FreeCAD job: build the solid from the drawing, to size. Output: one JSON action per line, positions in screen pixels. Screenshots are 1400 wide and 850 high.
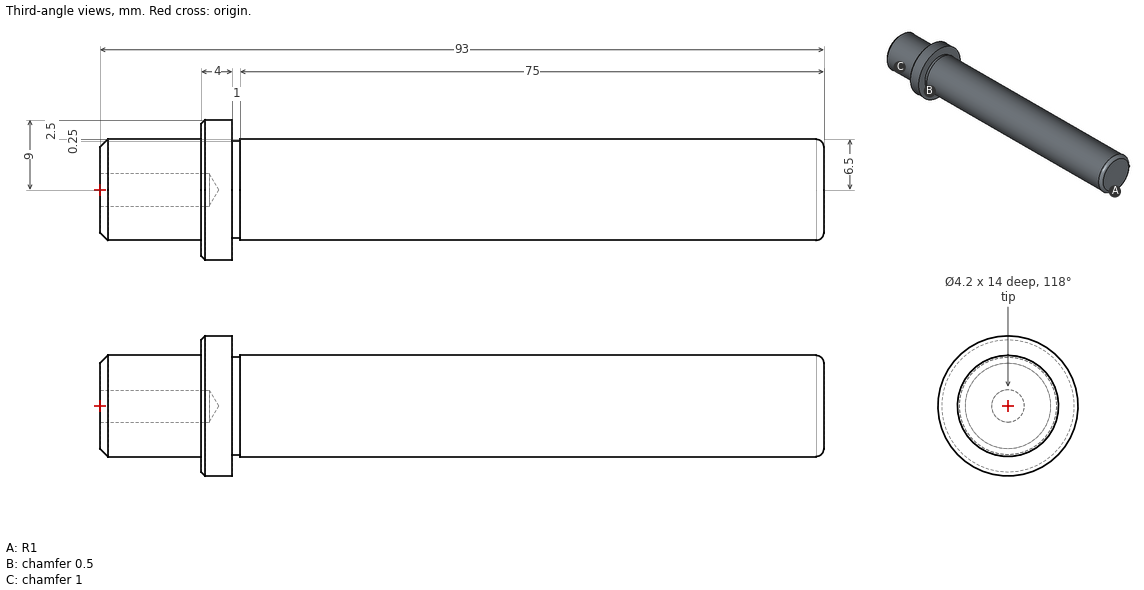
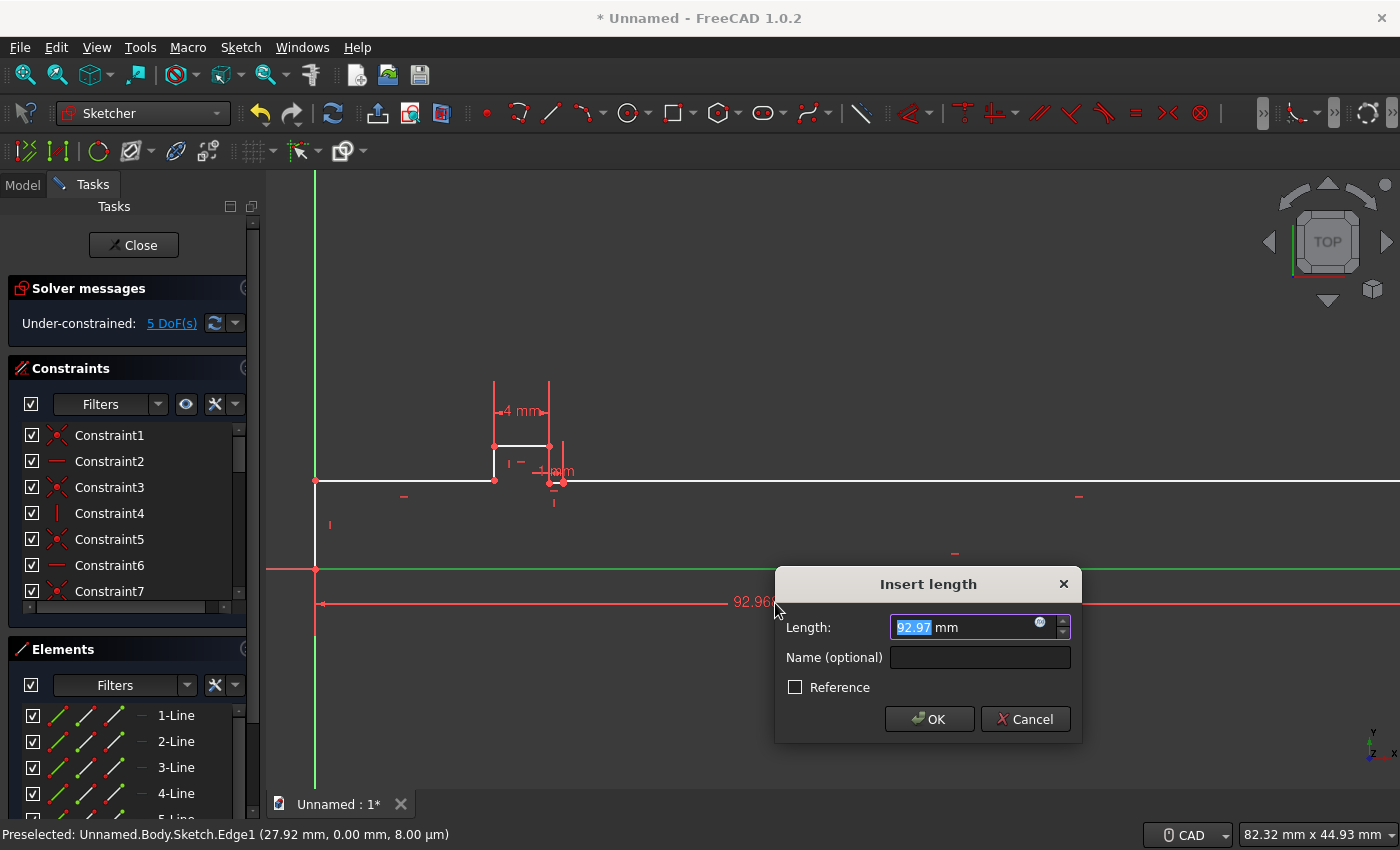
{"action": "type", "text": "93"}
{"action": "key", "text": "Return"}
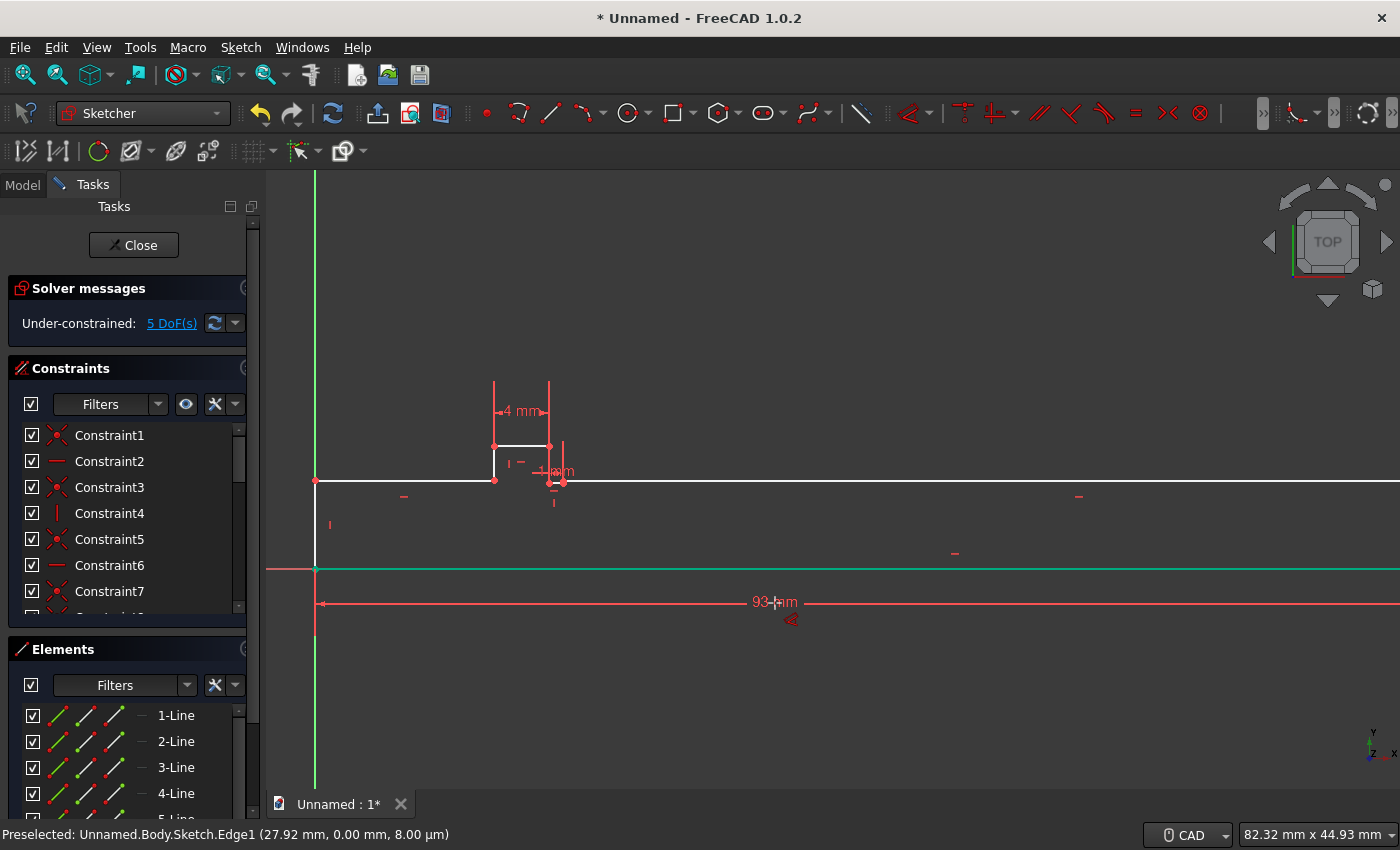
{"action": "left_click", "coordinate": [873, 481]}
{"action": "left_click", "coordinate": [899, 447]}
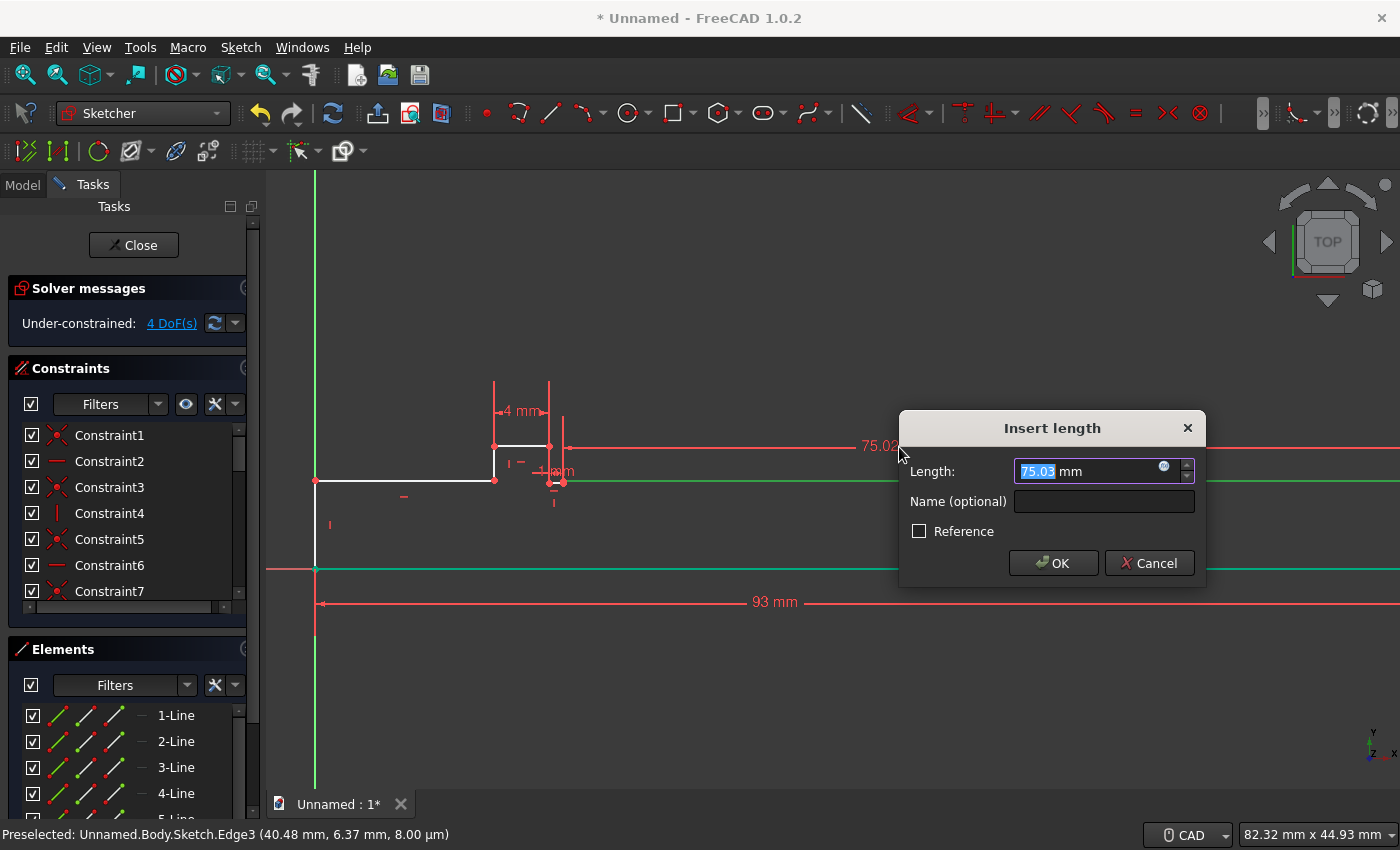
{"action": "type", "text": "75"}
{"action": "key", "text": "Return"}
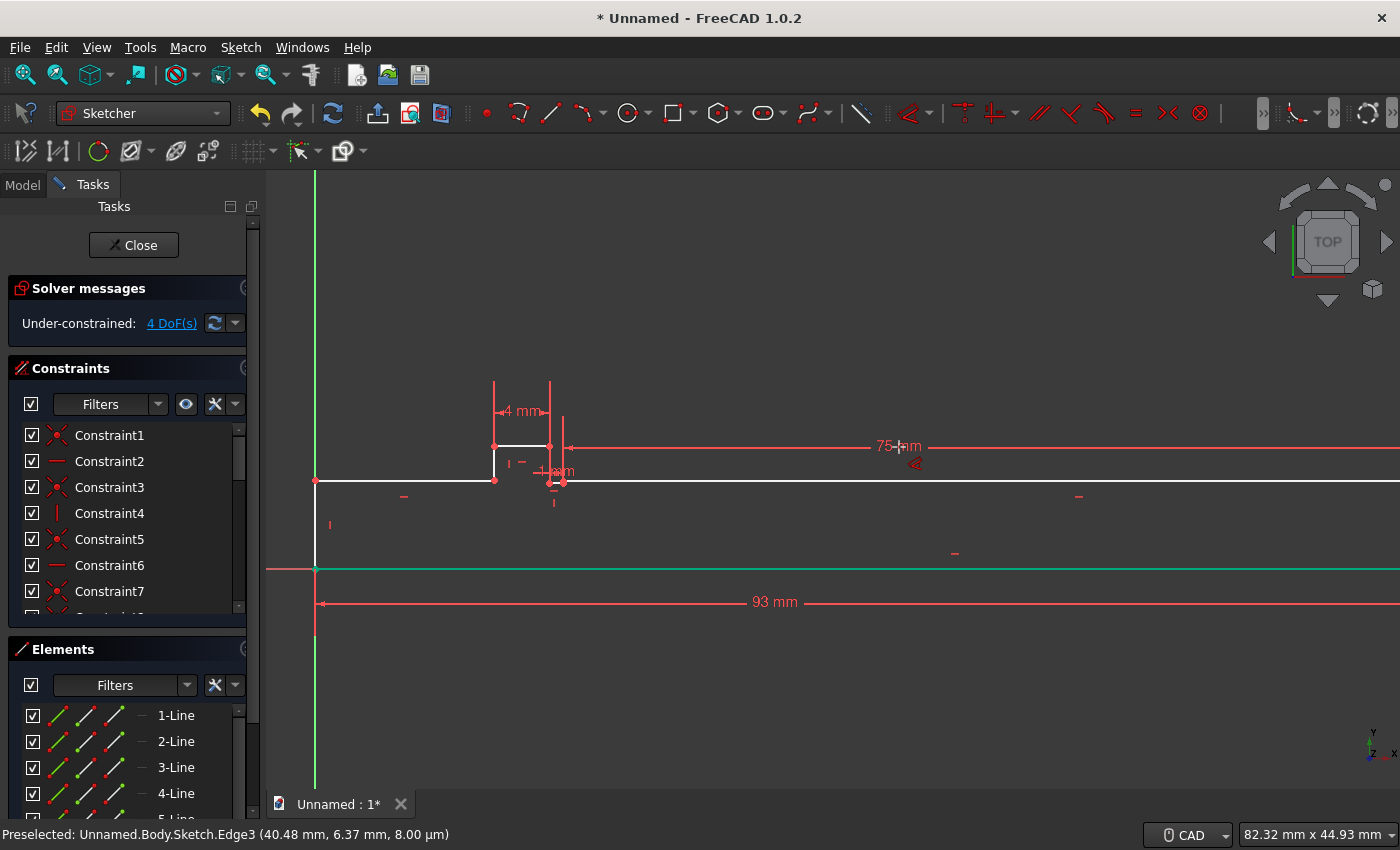
{"action": "left_click", "coordinate": [550, 446]}
{"action": "left_click", "coordinate": [584, 508]}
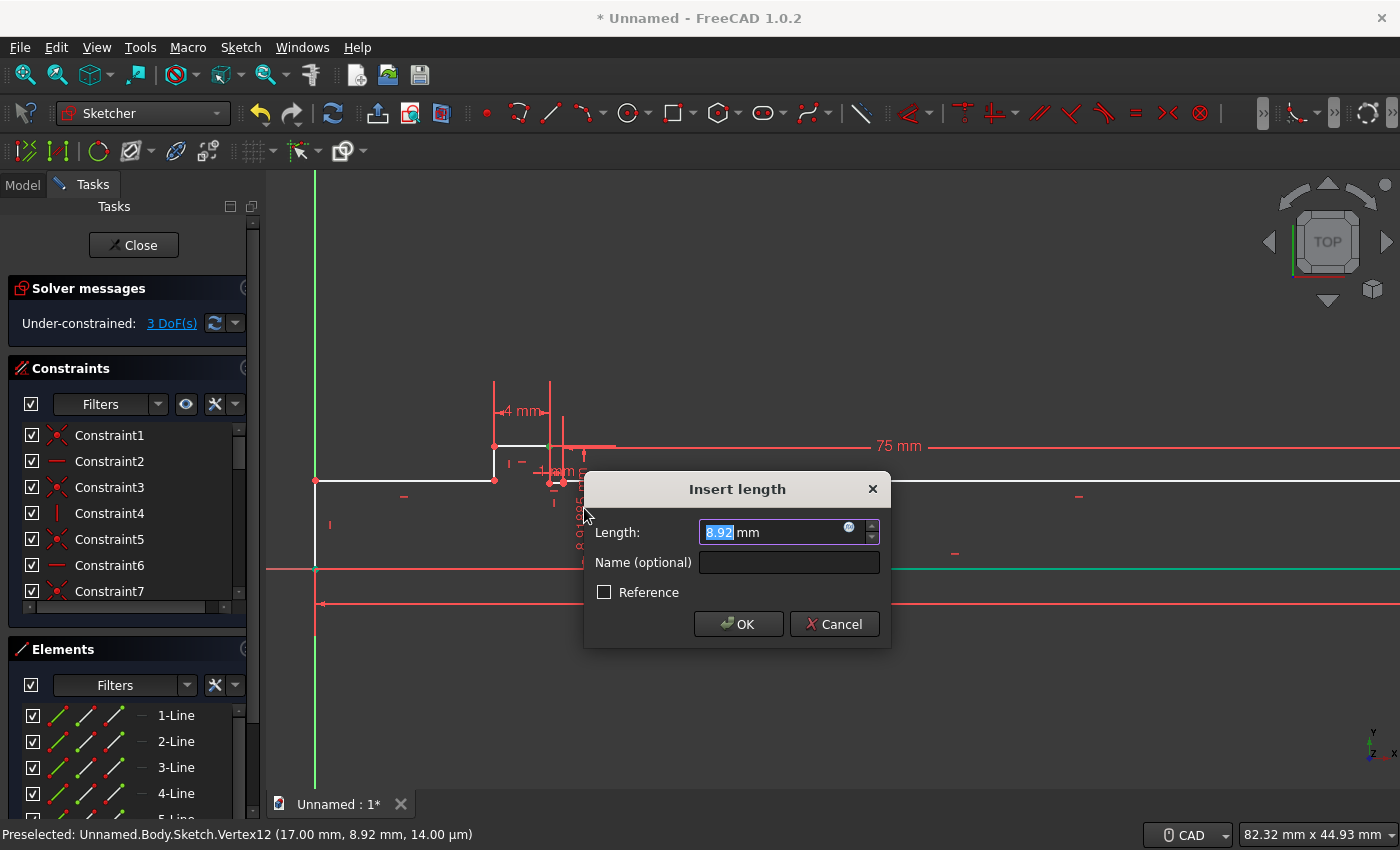
{"action": "type", "text": "9"}
{"action": "key", "text": "Return"}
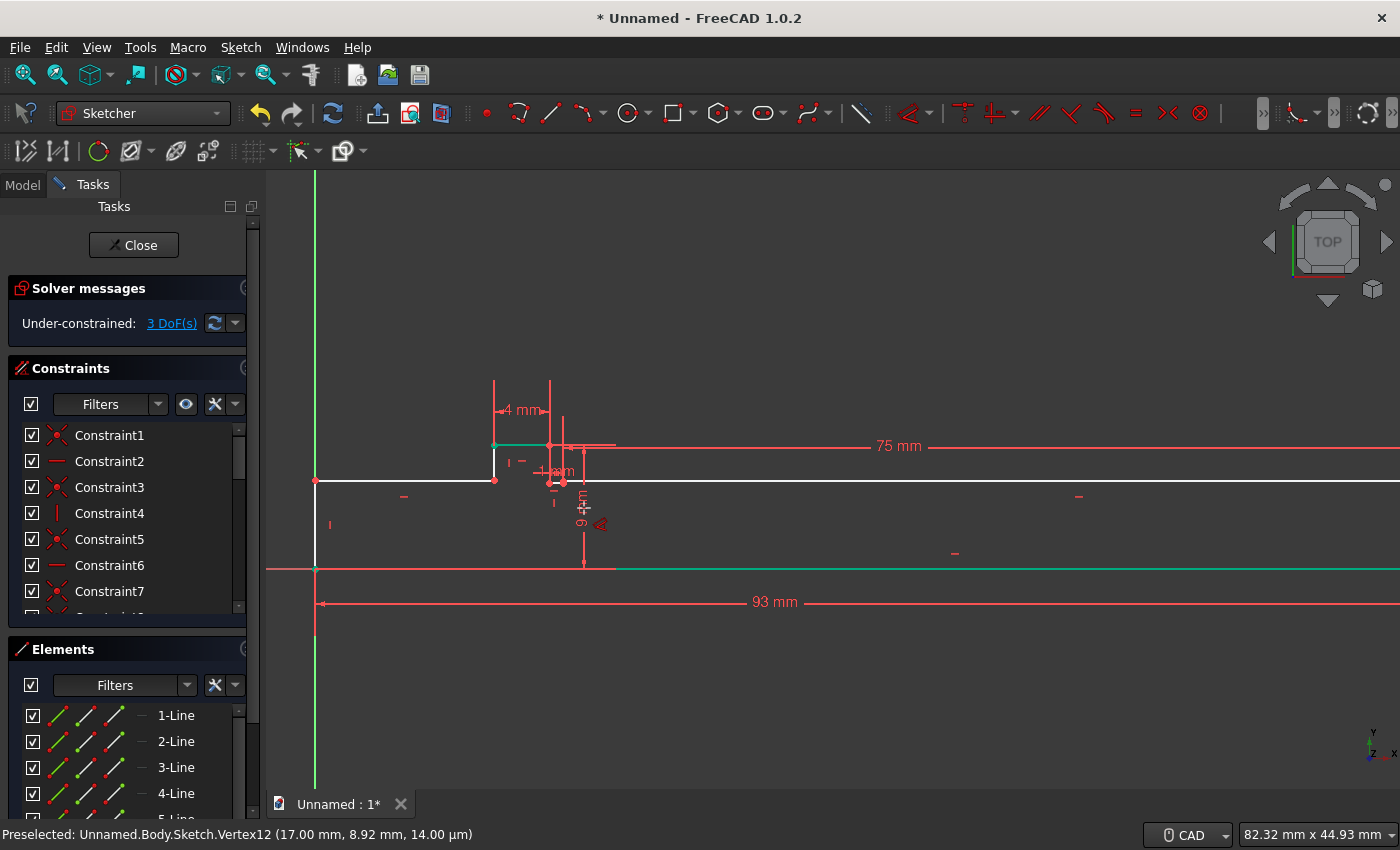
{"action": "scroll", "coordinate": [532, 446], "scroll_direction": "down", "scroll_amount": 3}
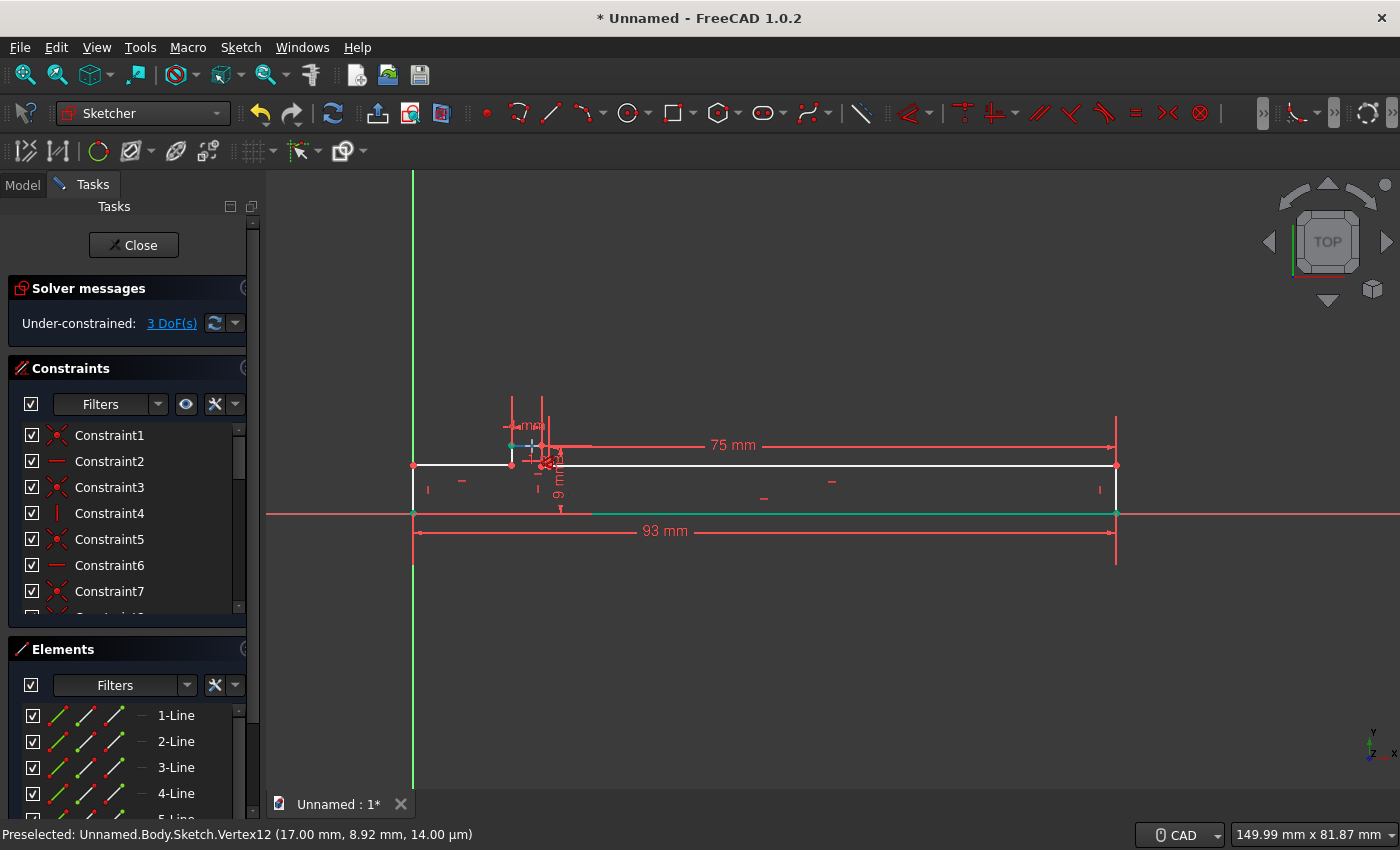
{"action": "left_click", "coordinate": [1116, 499]}
{"action": "left_click", "coordinate": [1150, 490]}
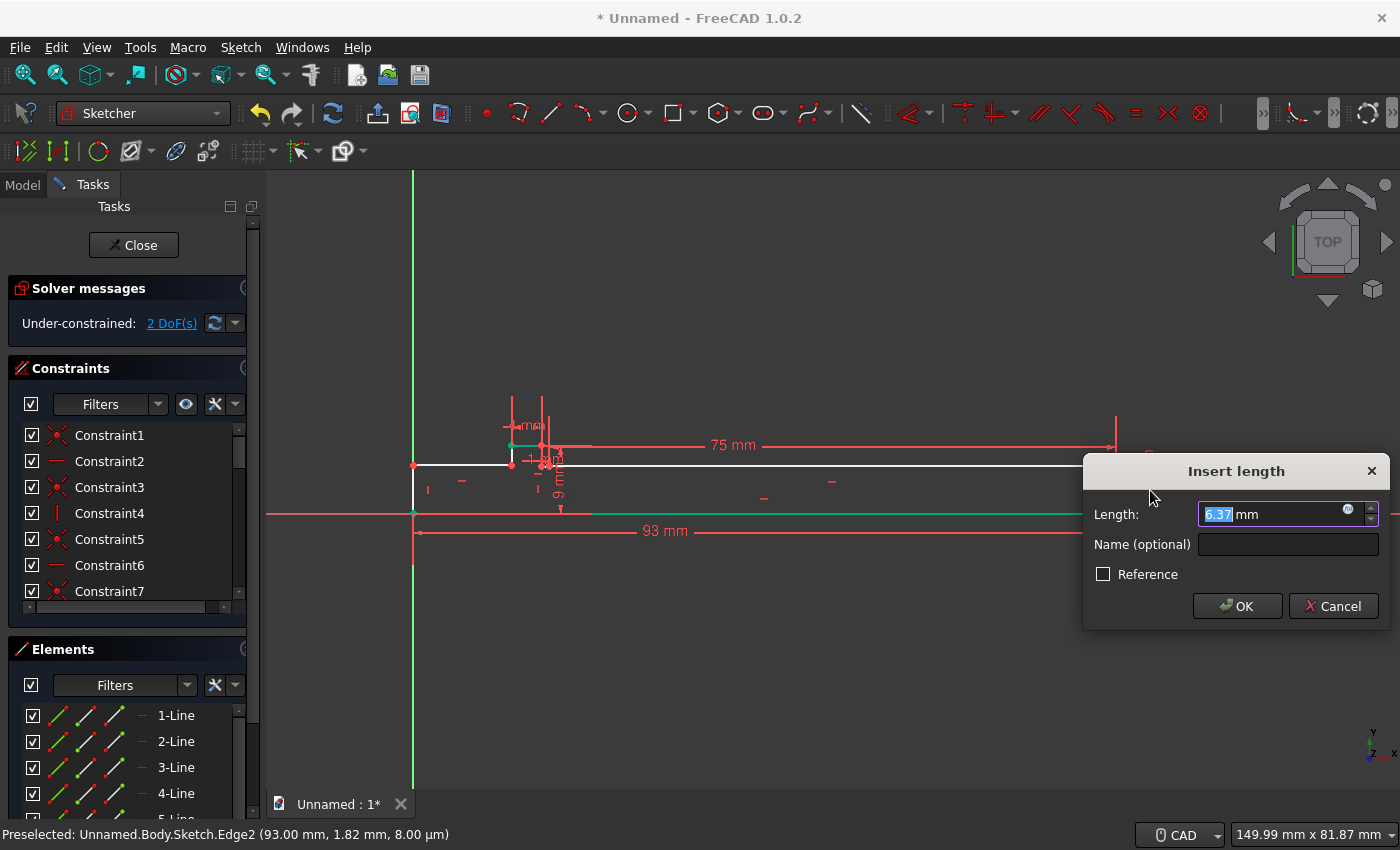
{"action": "type", "text": "6.5"}
{"action": "key", "text": "Return"}